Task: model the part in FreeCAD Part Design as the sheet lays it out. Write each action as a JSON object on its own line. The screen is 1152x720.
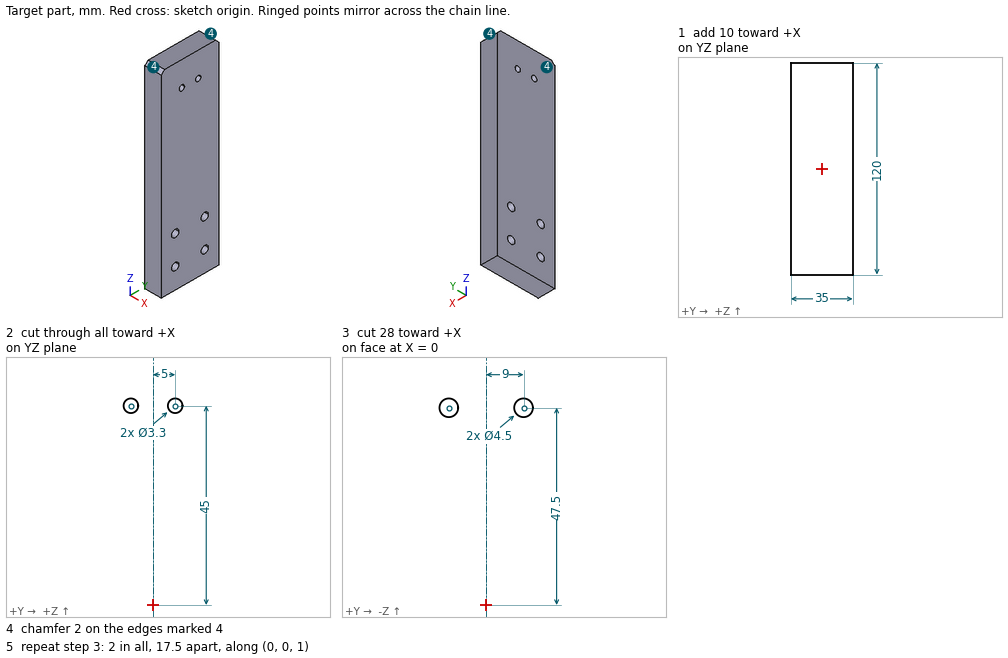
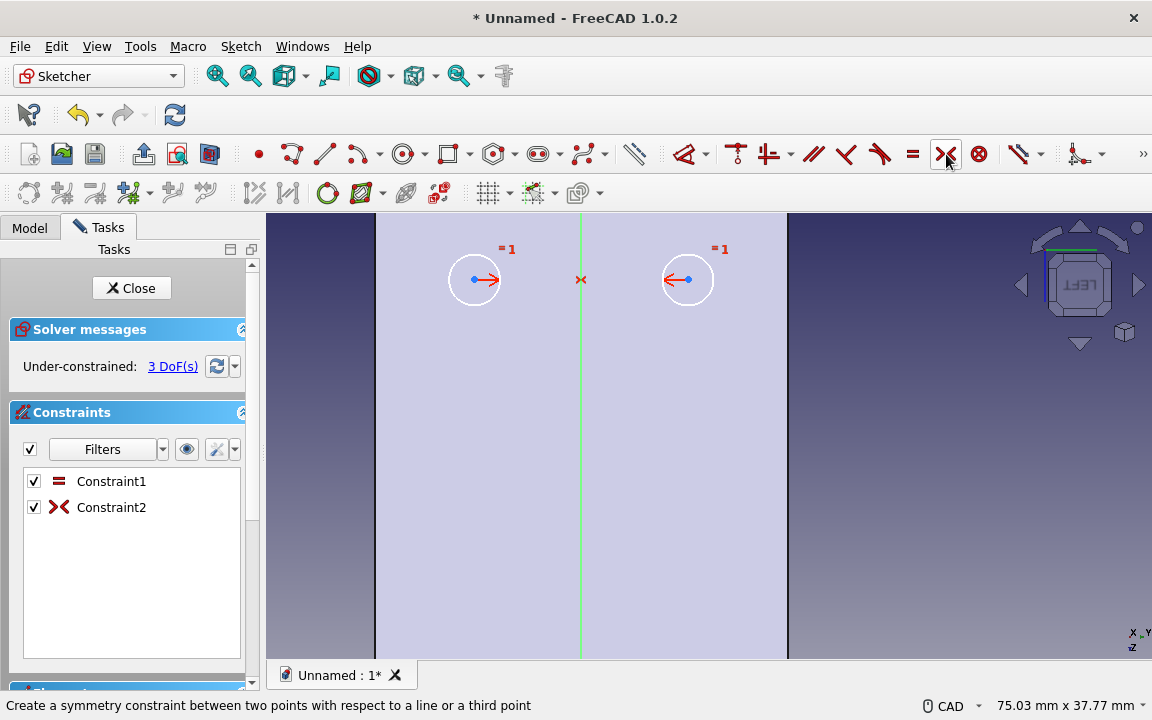
{"action": "left_click", "coordinate": [684, 154]}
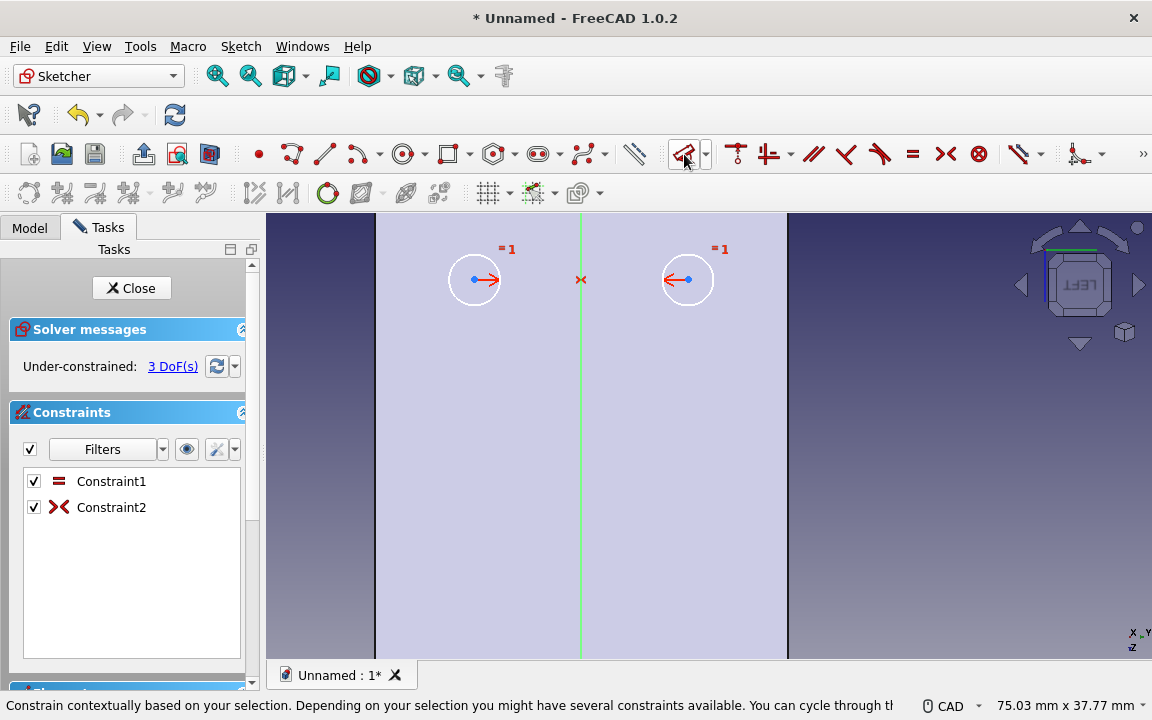
{"action": "left_click", "coordinate": [706, 262]}
{"action": "left_click", "coordinate": [743, 264]}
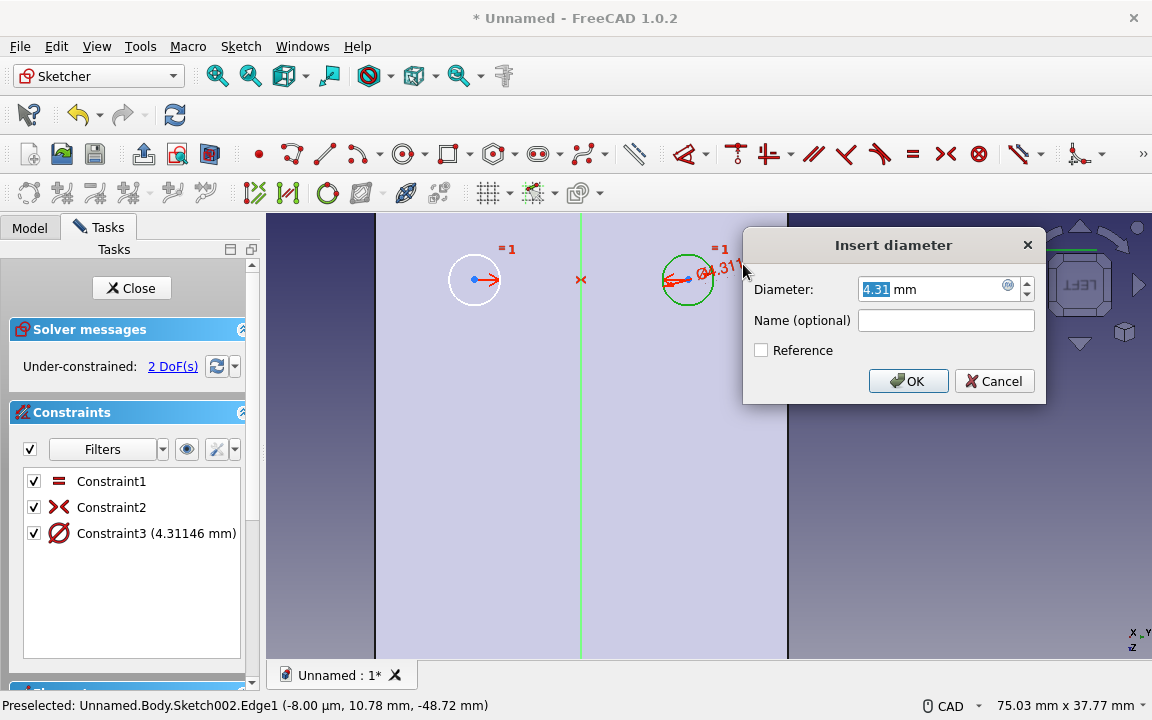
{"action": "type", "text": "4.5"}
{"action": "key", "text": "Return"}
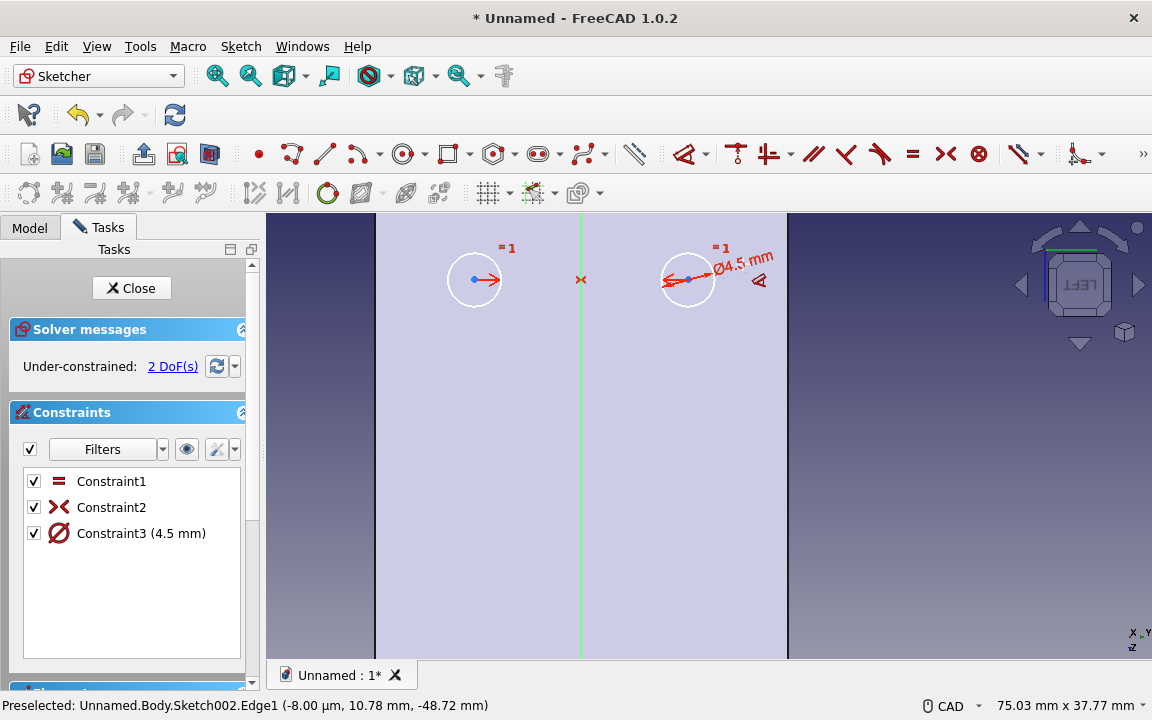
{"action": "left_click", "coordinate": [688, 280]}
{"action": "left_click", "coordinate": [635, 246]}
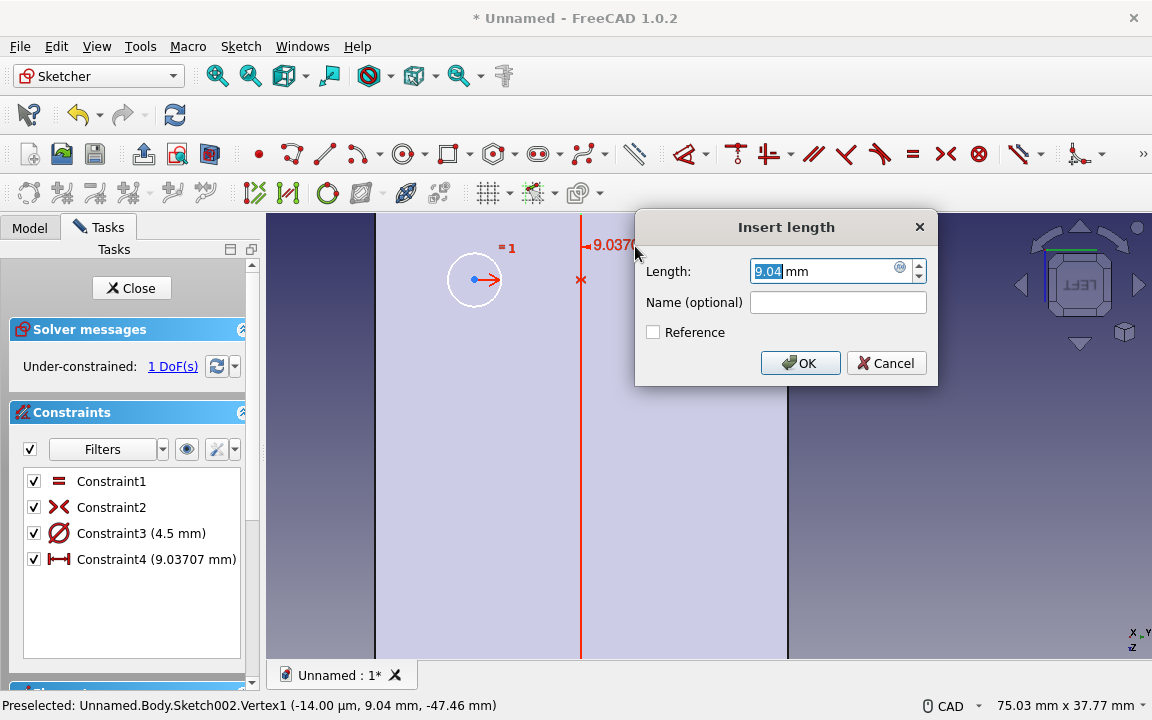
{"action": "type", "text": "9"}
{"action": "key", "text": "Return"}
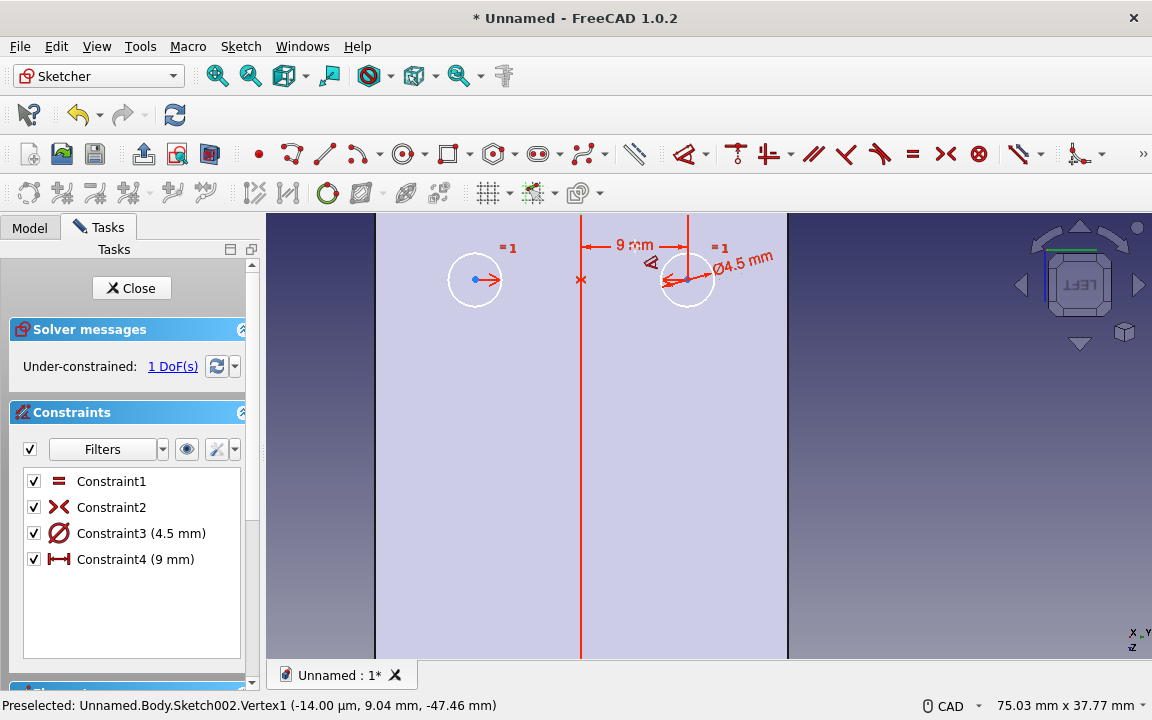
{"action": "left_click", "coordinate": [688, 280]}
{"action": "left_click", "coordinate": [722, 455]}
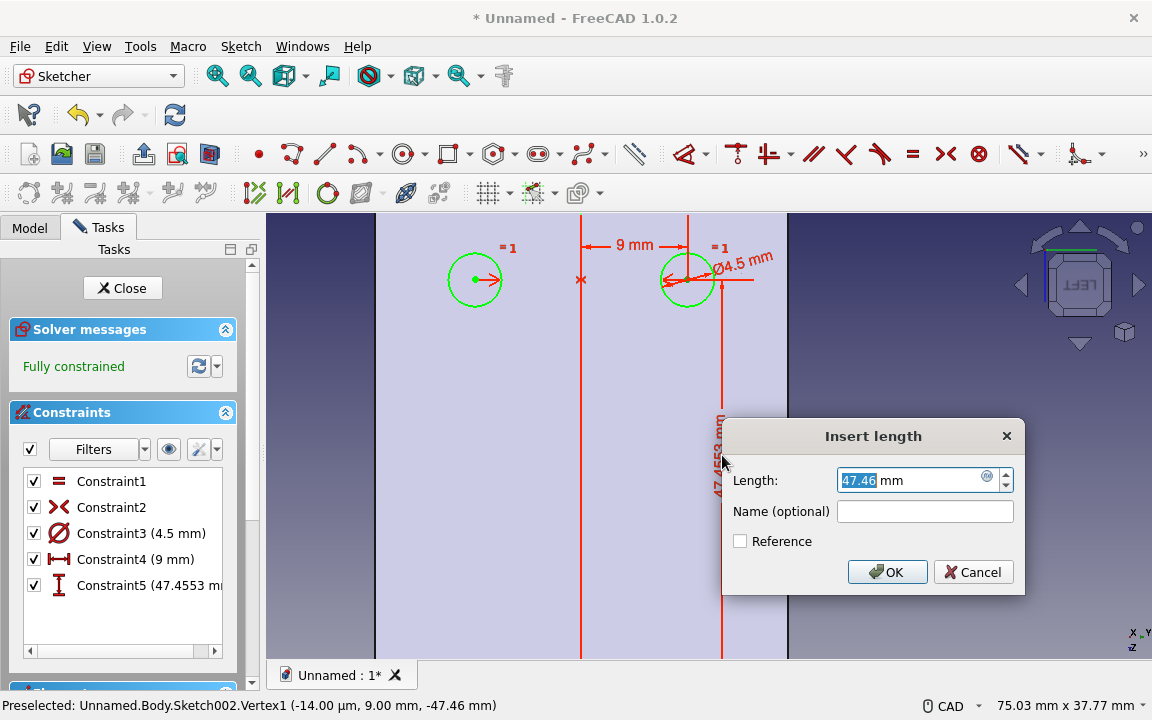
{"action": "type", "text": "47.5"}
{"action": "key", "text": "Return"}
{"action": "key", "text": "Escape"}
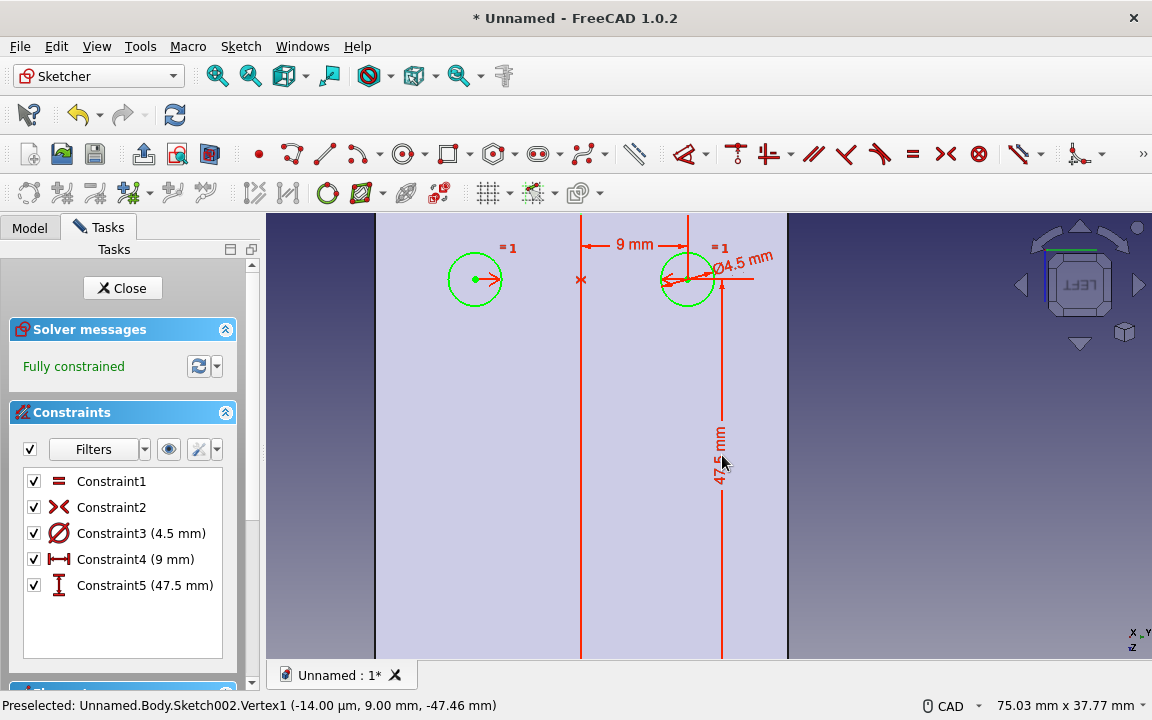
{"action": "left_click", "coordinate": [123, 288]}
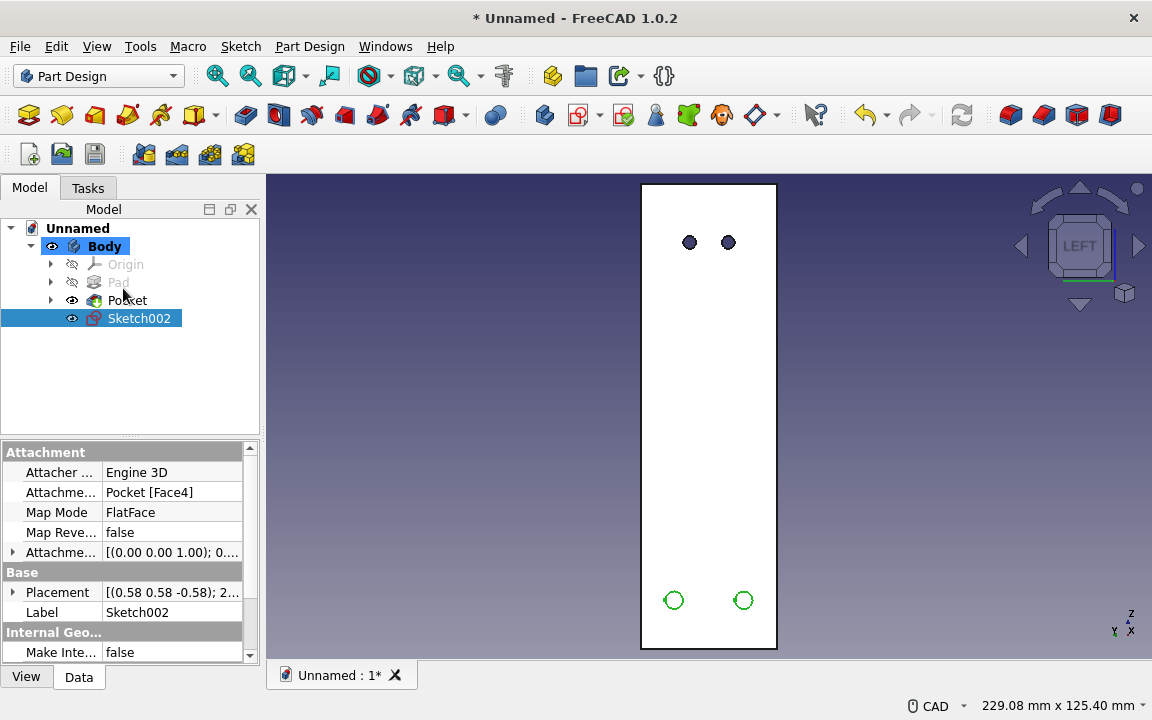
{"action": "left_click", "coordinate": [246, 116]}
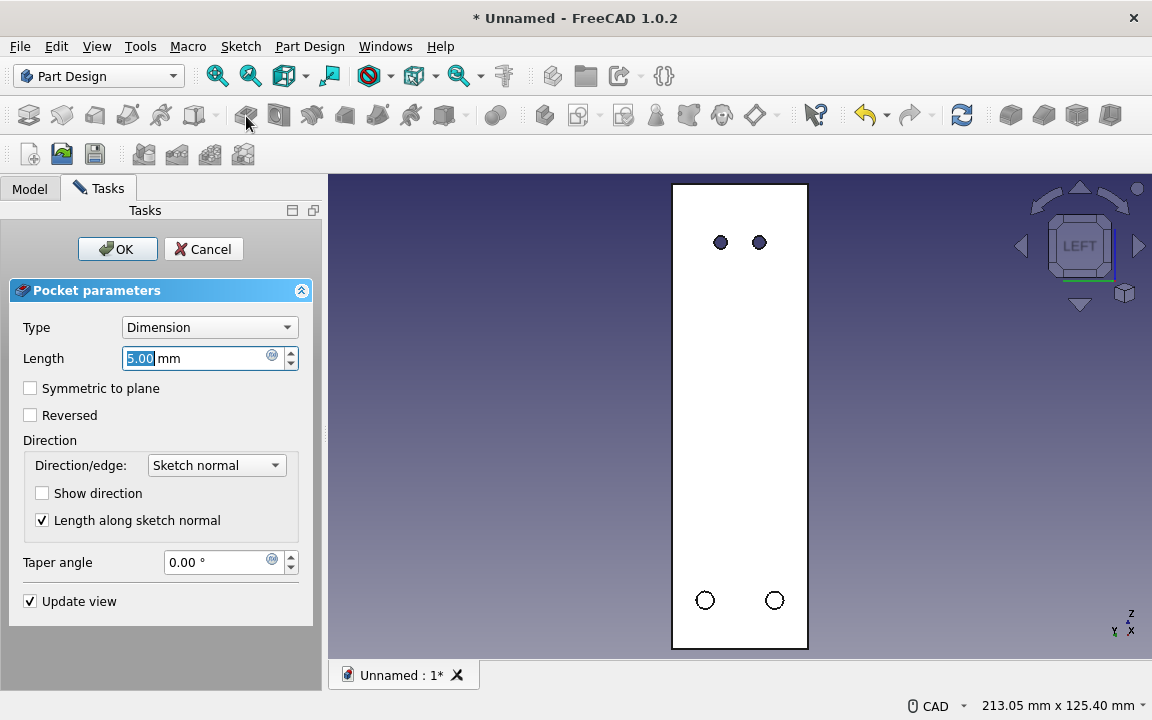
{"action": "type", "text": "28"}
{"action": "key", "text": "Tab"}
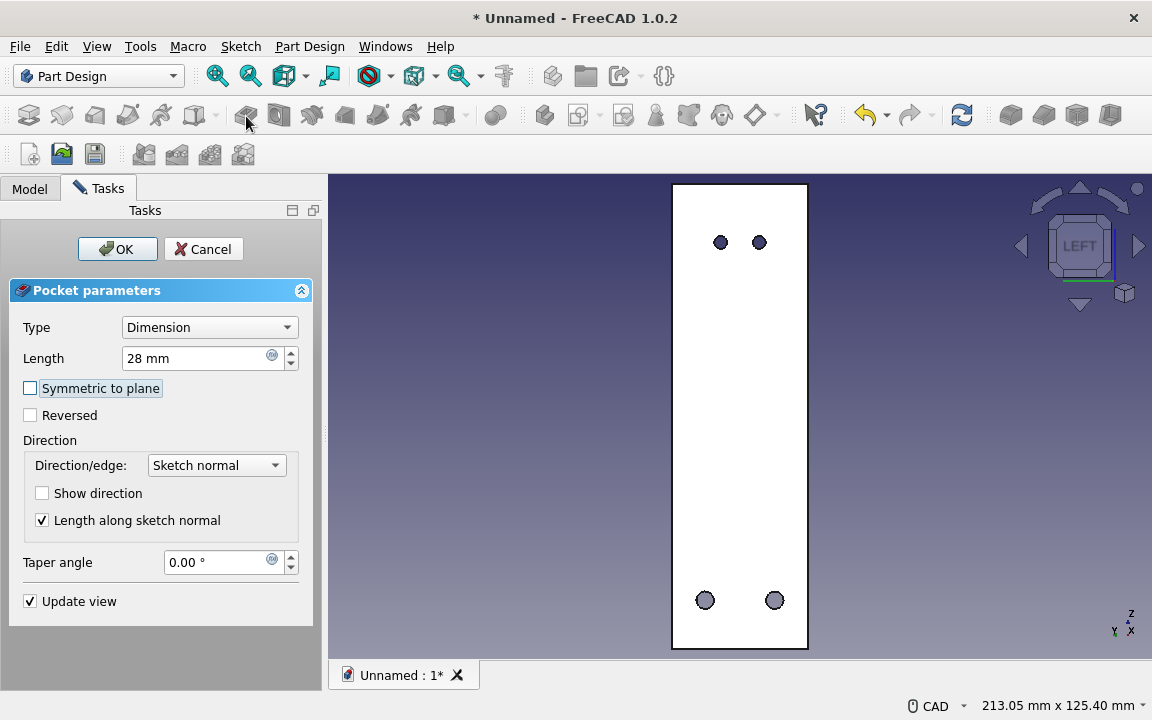
{"action": "left_click", "coordinate": [118, 249]}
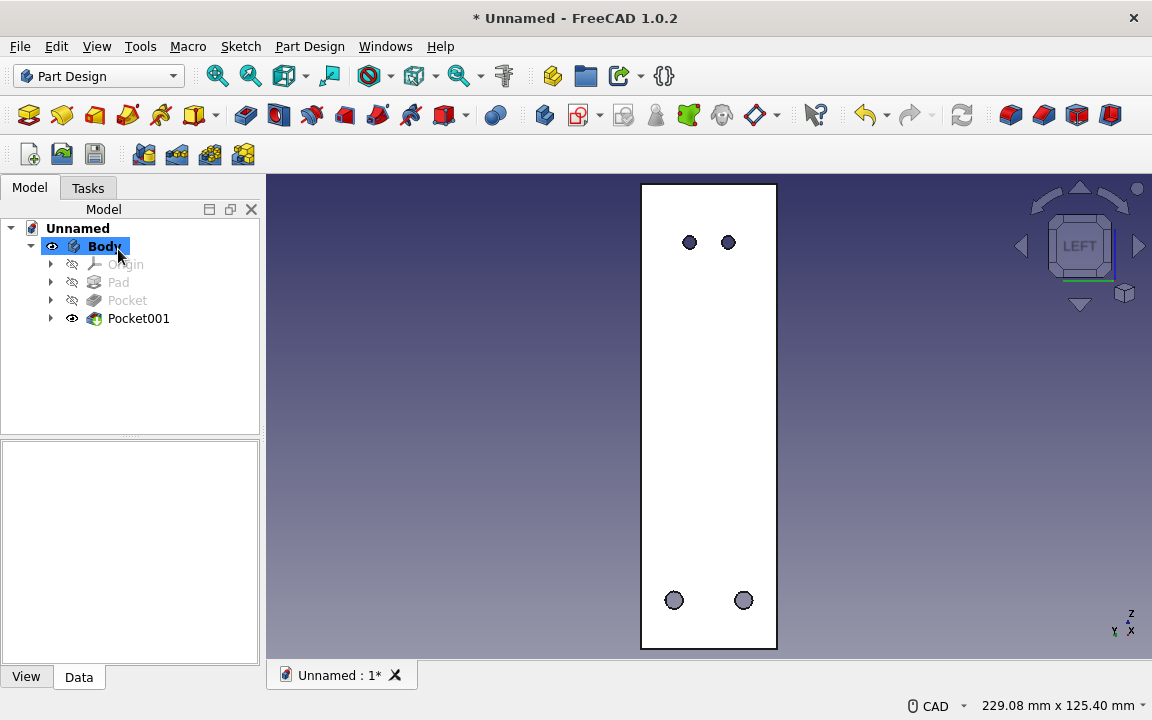
{"action": "key", "text": "0"}